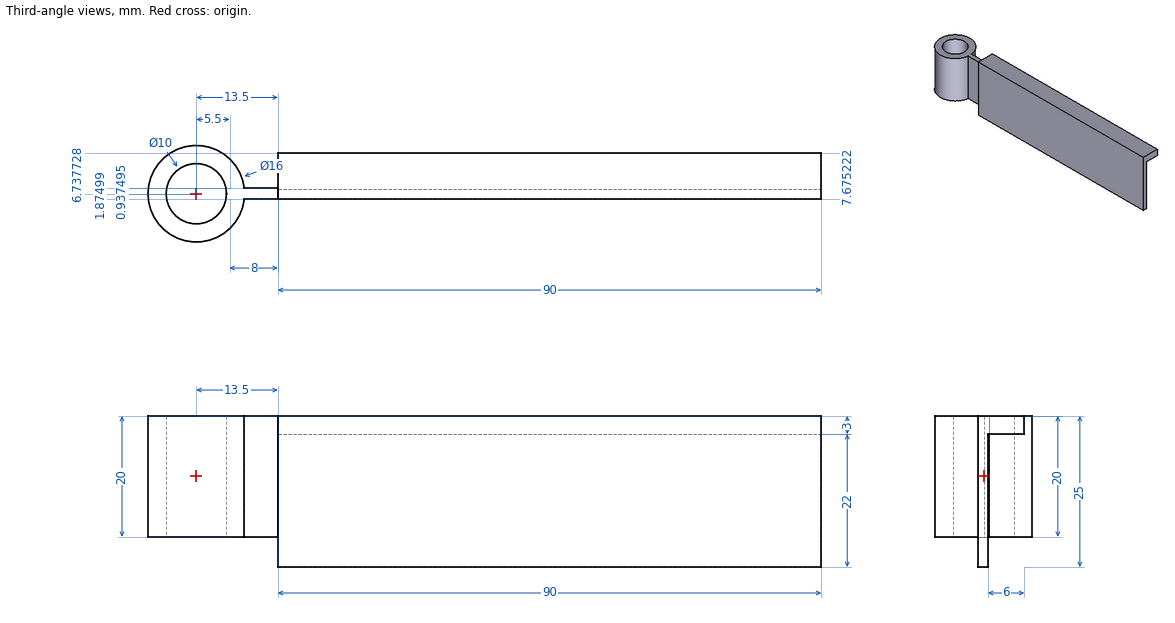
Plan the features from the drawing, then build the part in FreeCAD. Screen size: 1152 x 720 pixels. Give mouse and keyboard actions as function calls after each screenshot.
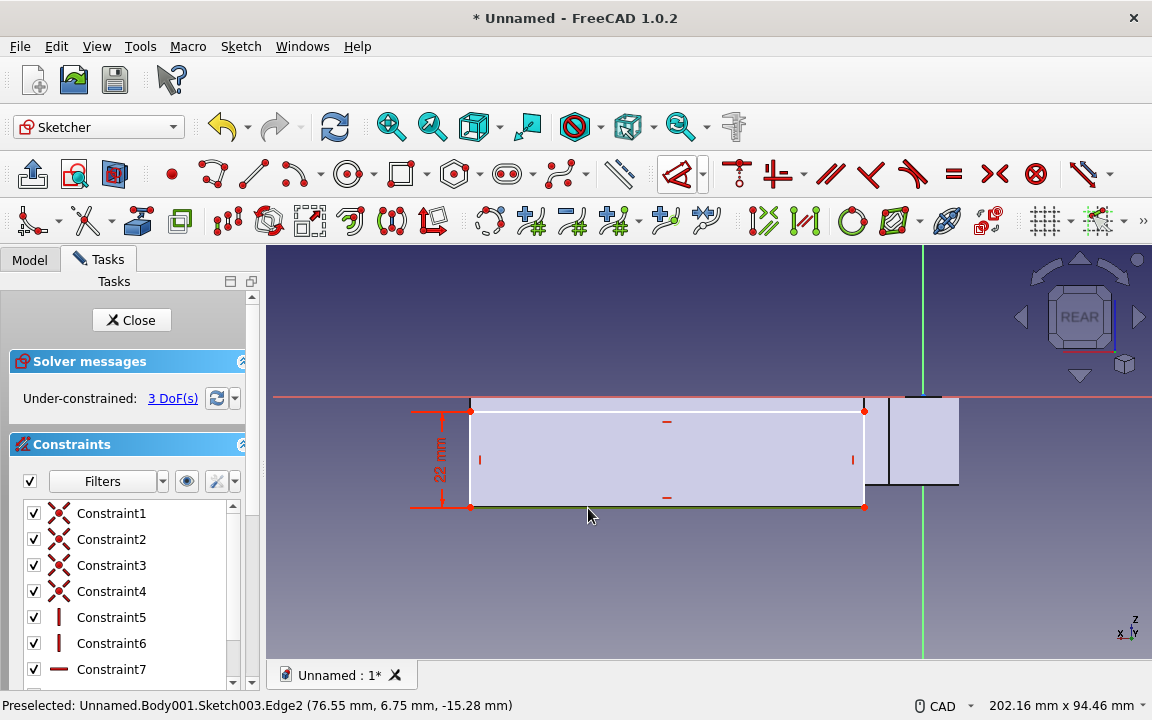
key(l)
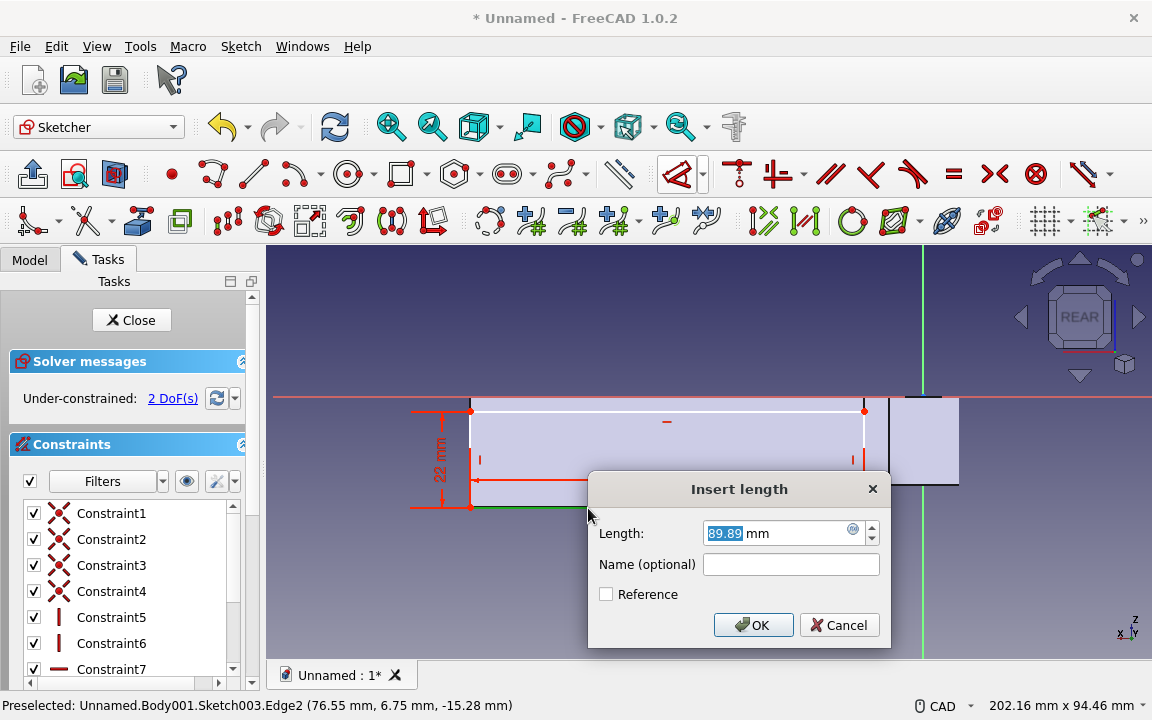
text(90)
key(Return)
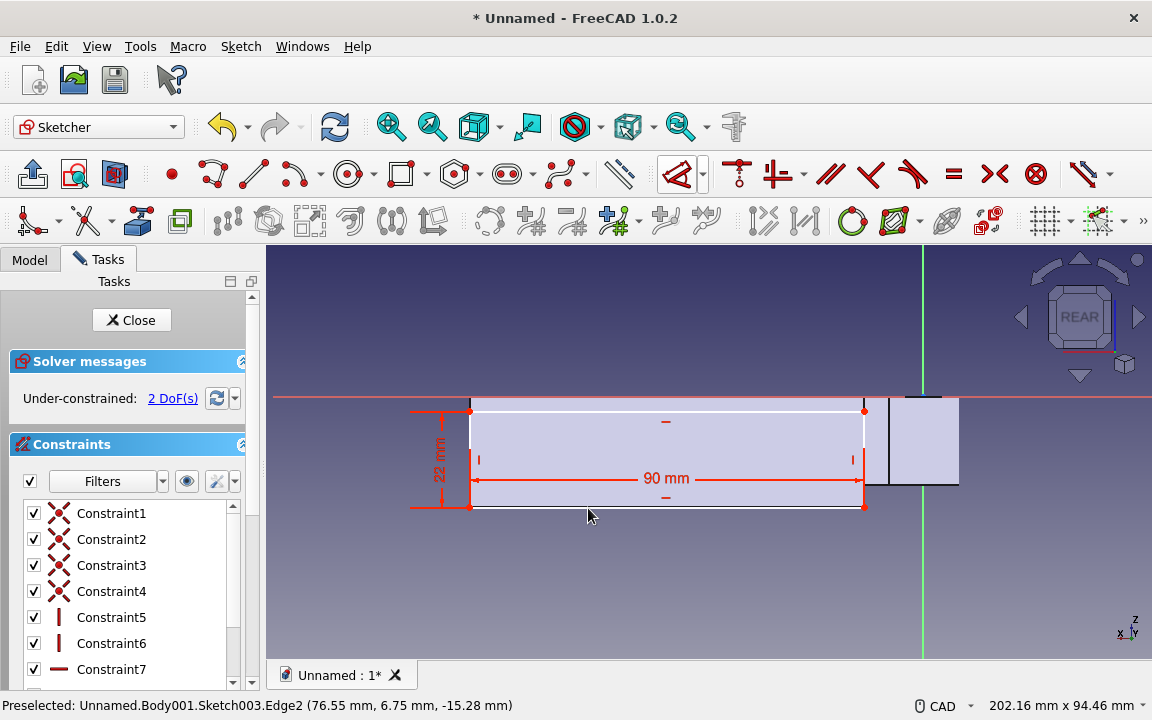
scroll(470, 412, up, 6)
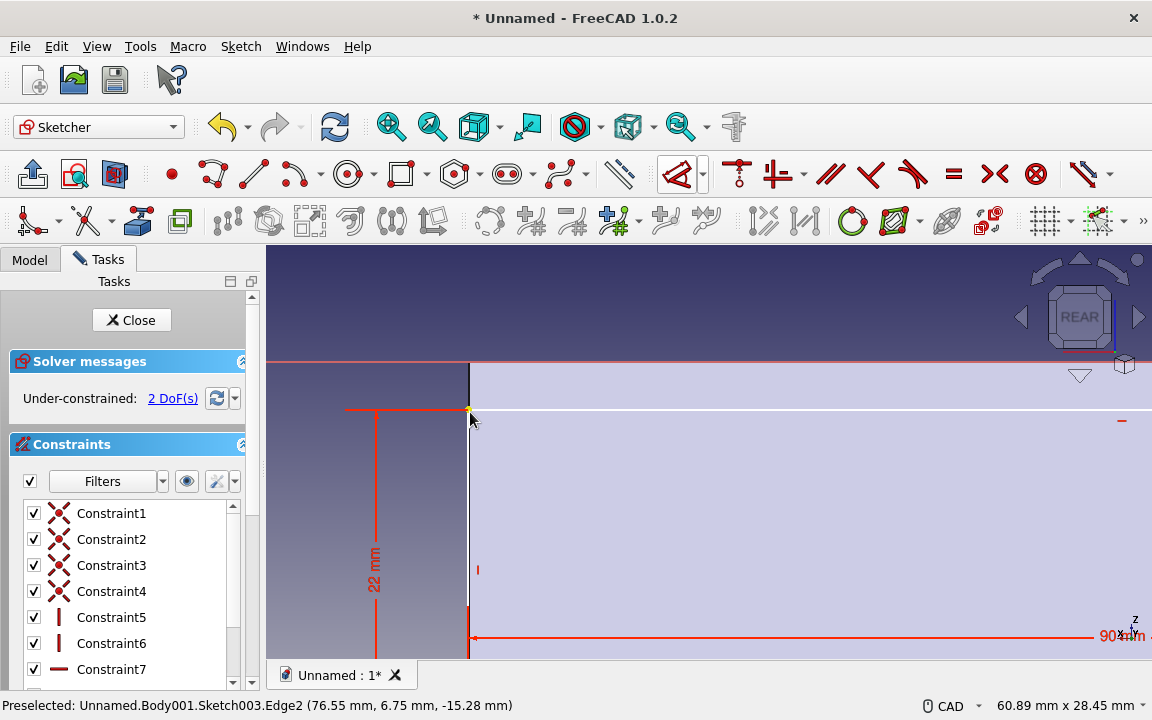
click(468, 410)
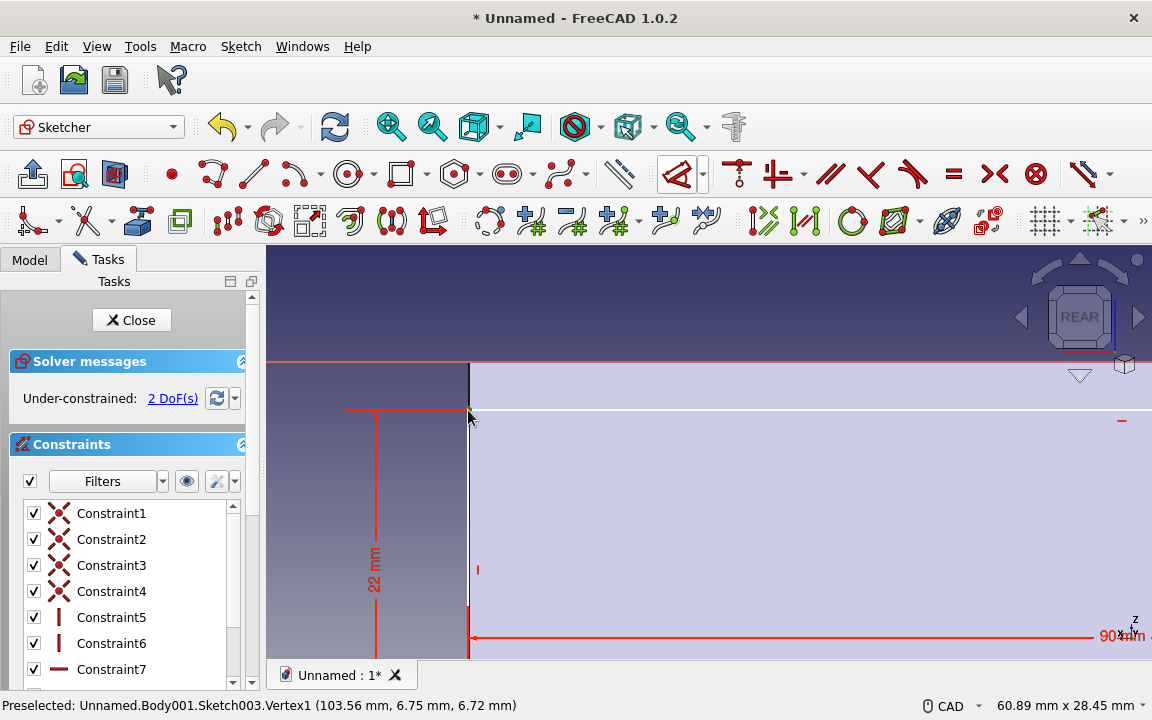
click(702, 174)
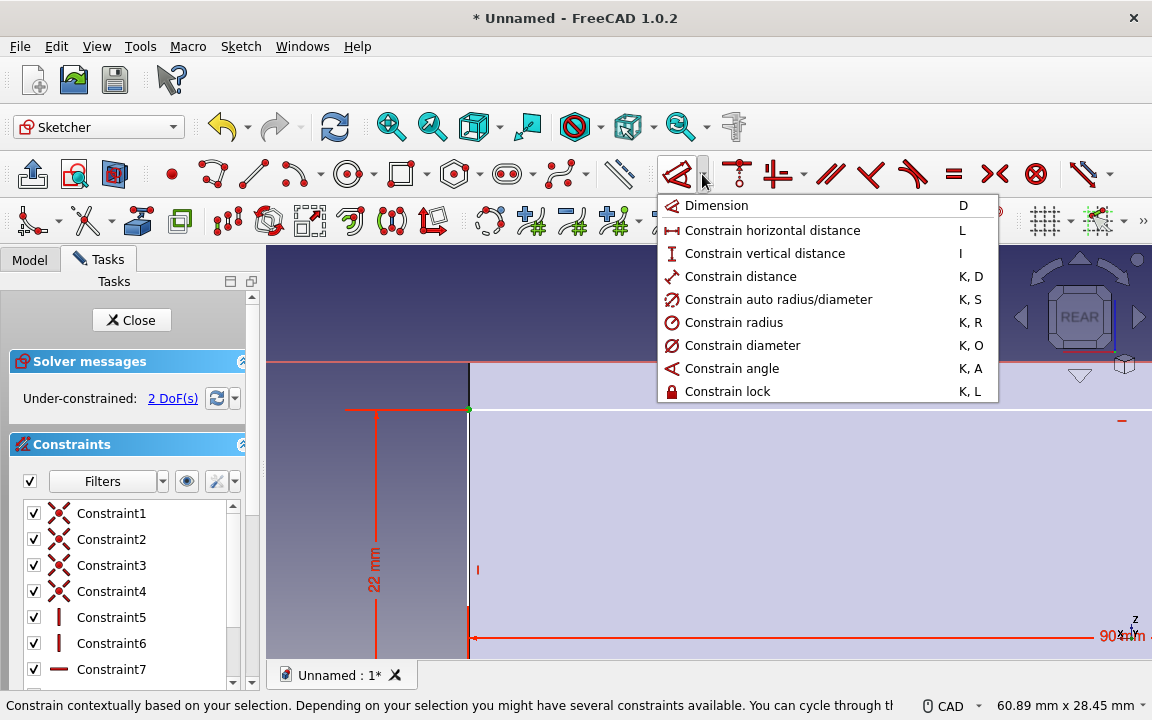
click(828, 254)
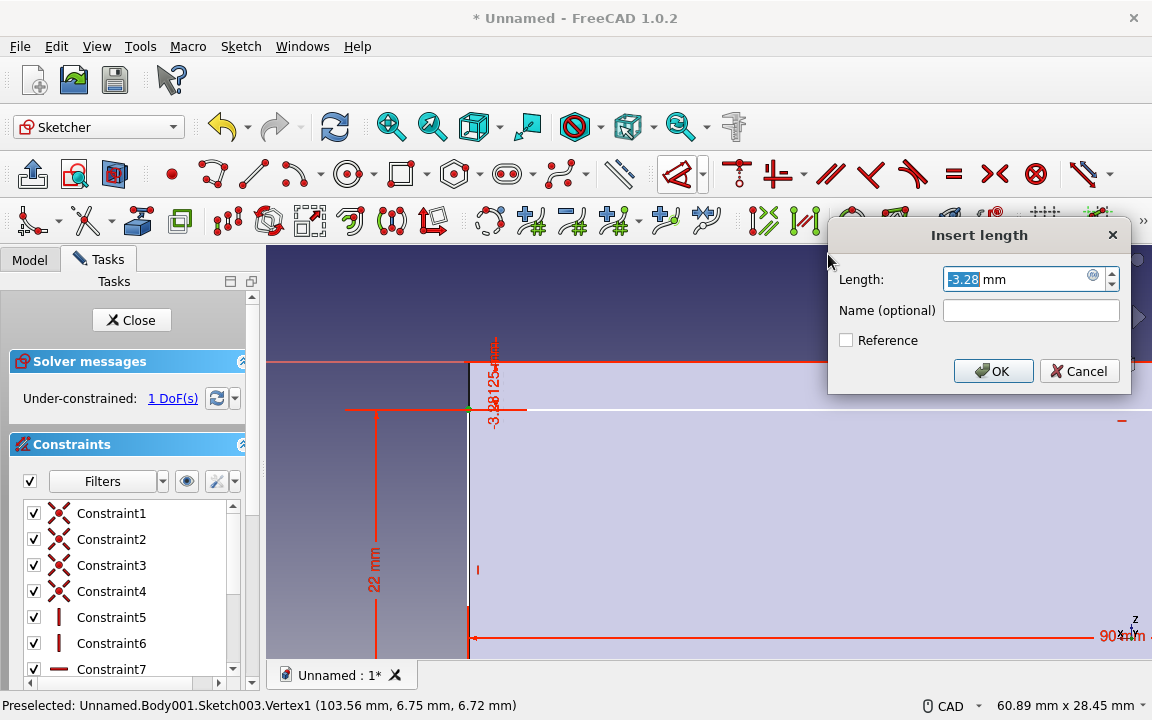
text(-3)
key(Return)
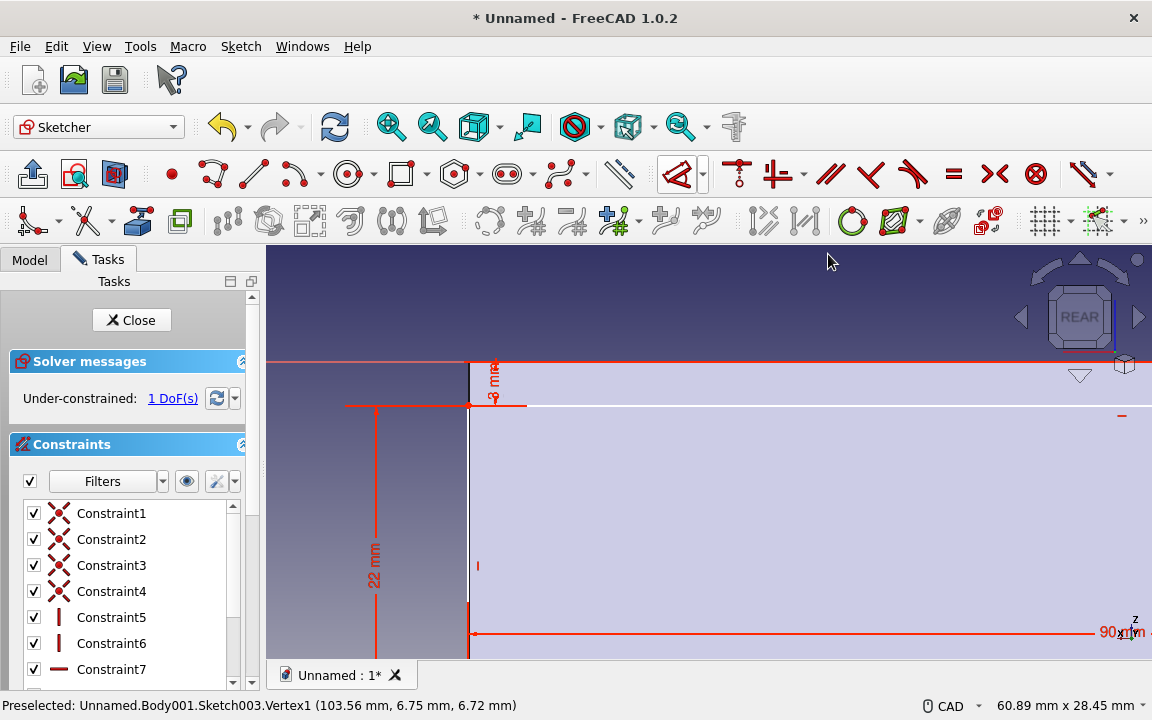
scroll(390, 412, down, 6)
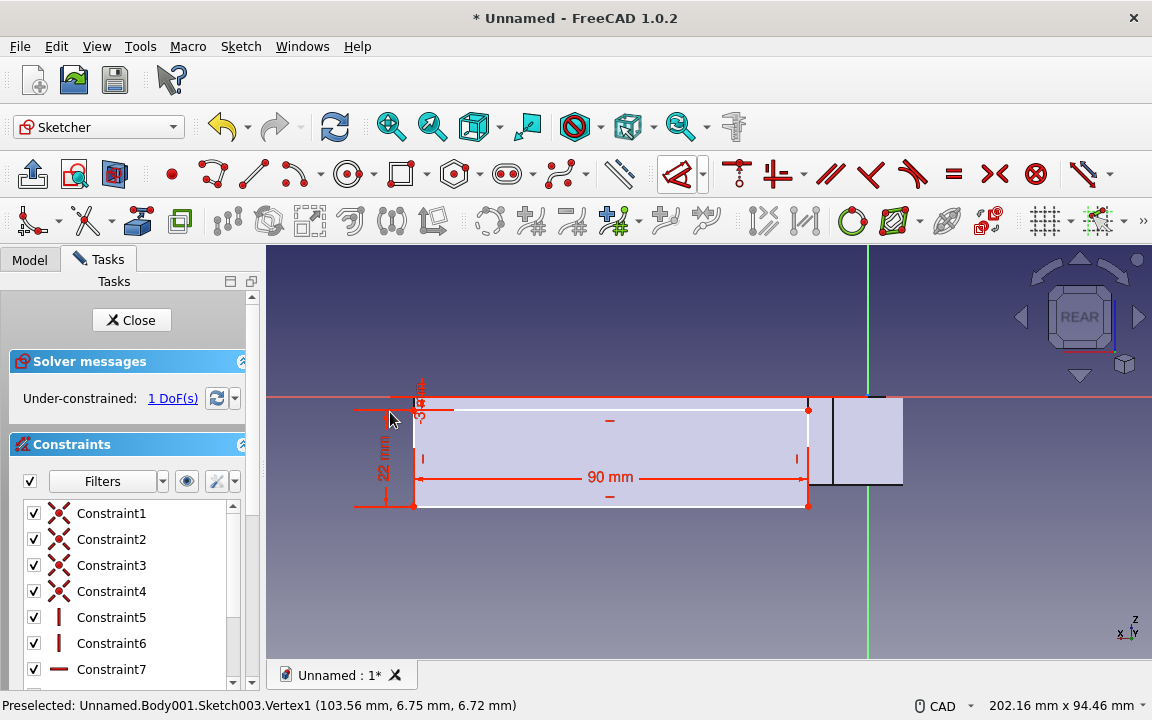
click(808, 507)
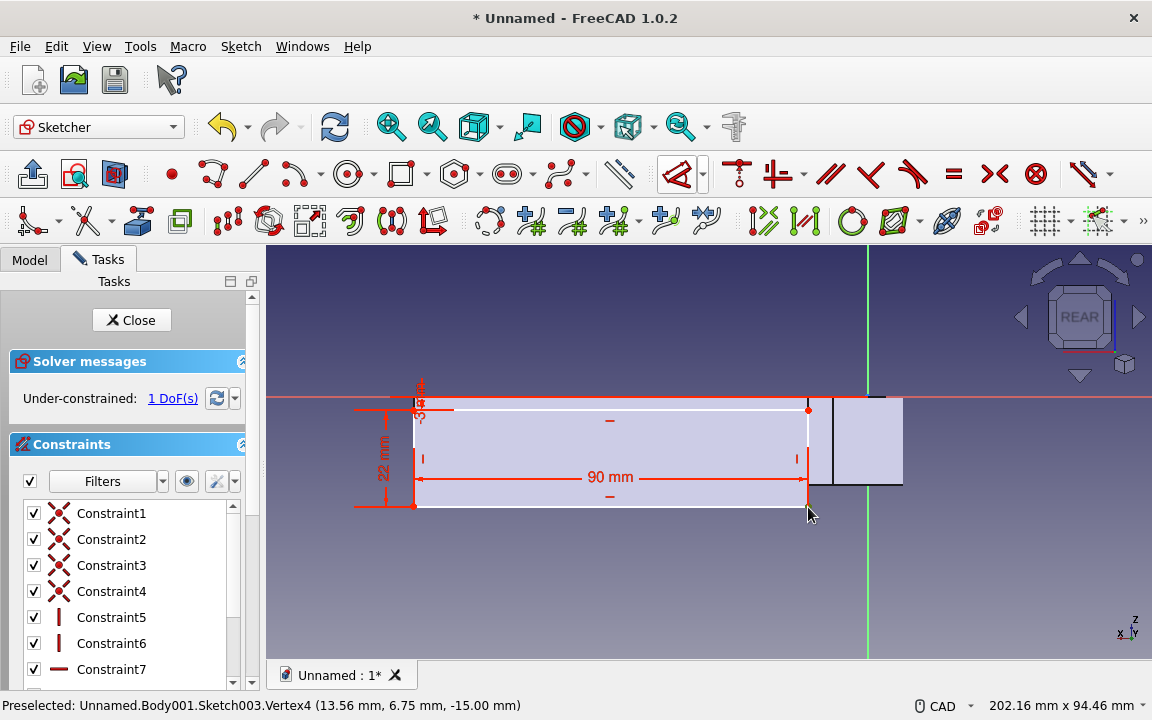
click(702, 174)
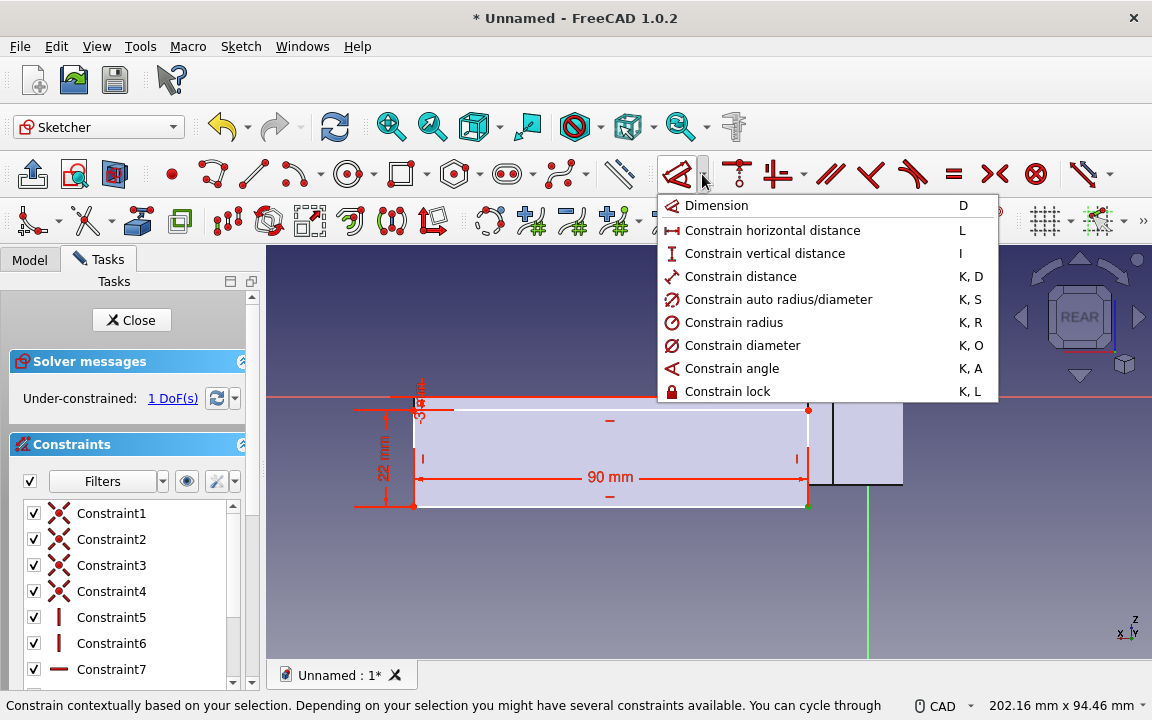
click(828, 230)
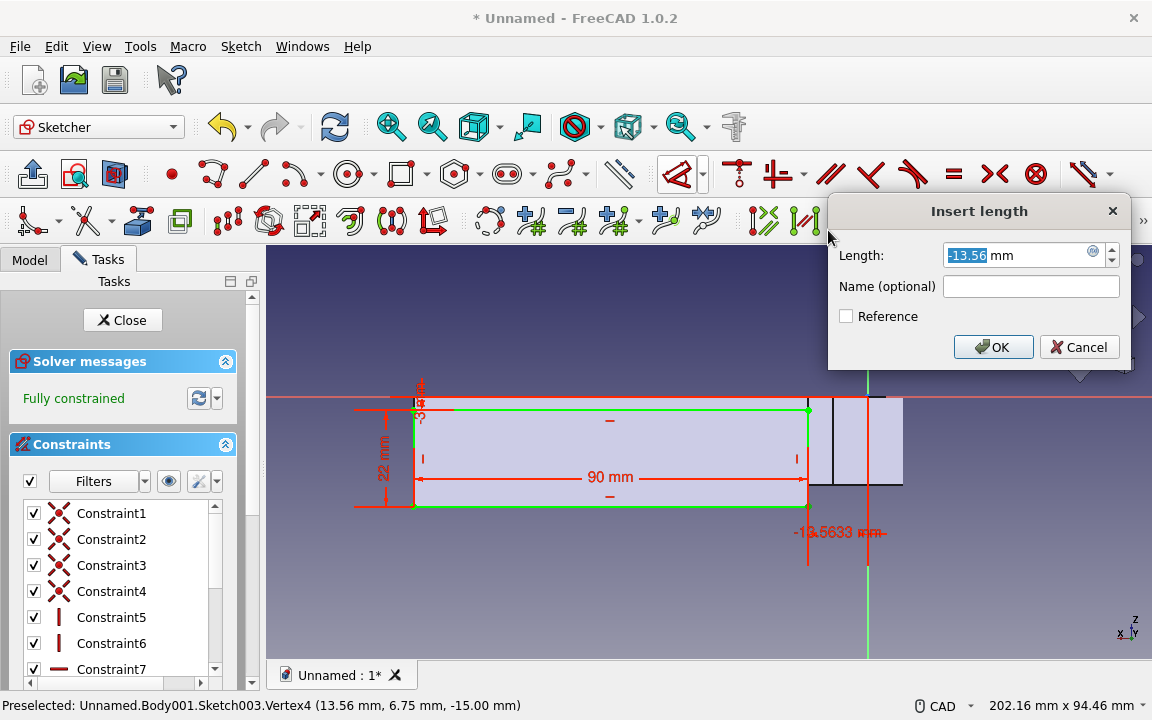
text(-13.5)
key(Return)